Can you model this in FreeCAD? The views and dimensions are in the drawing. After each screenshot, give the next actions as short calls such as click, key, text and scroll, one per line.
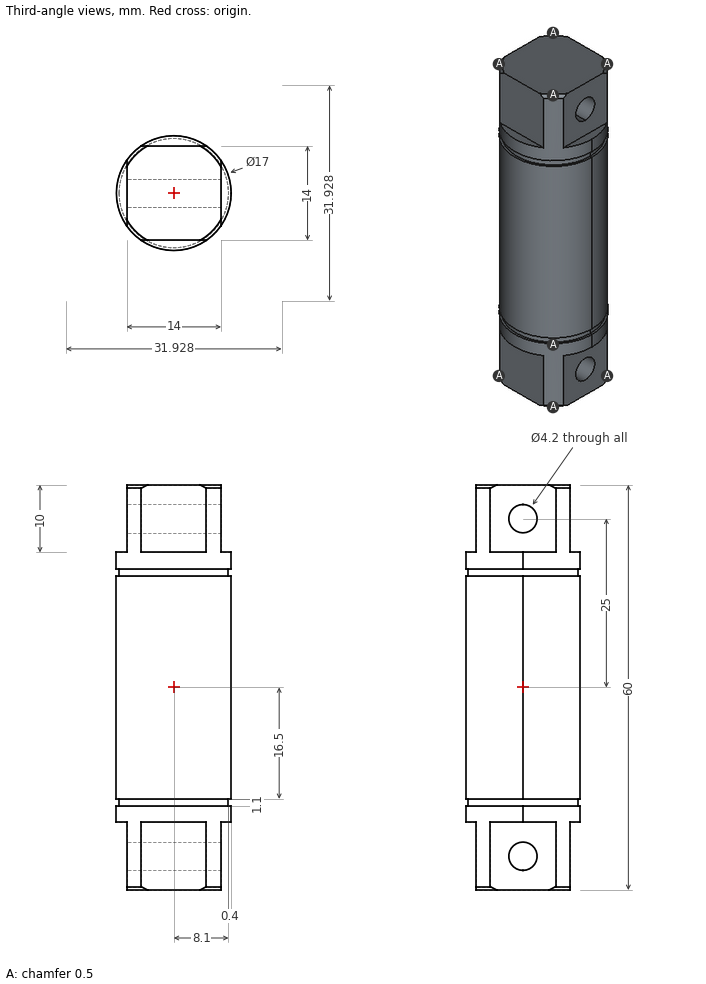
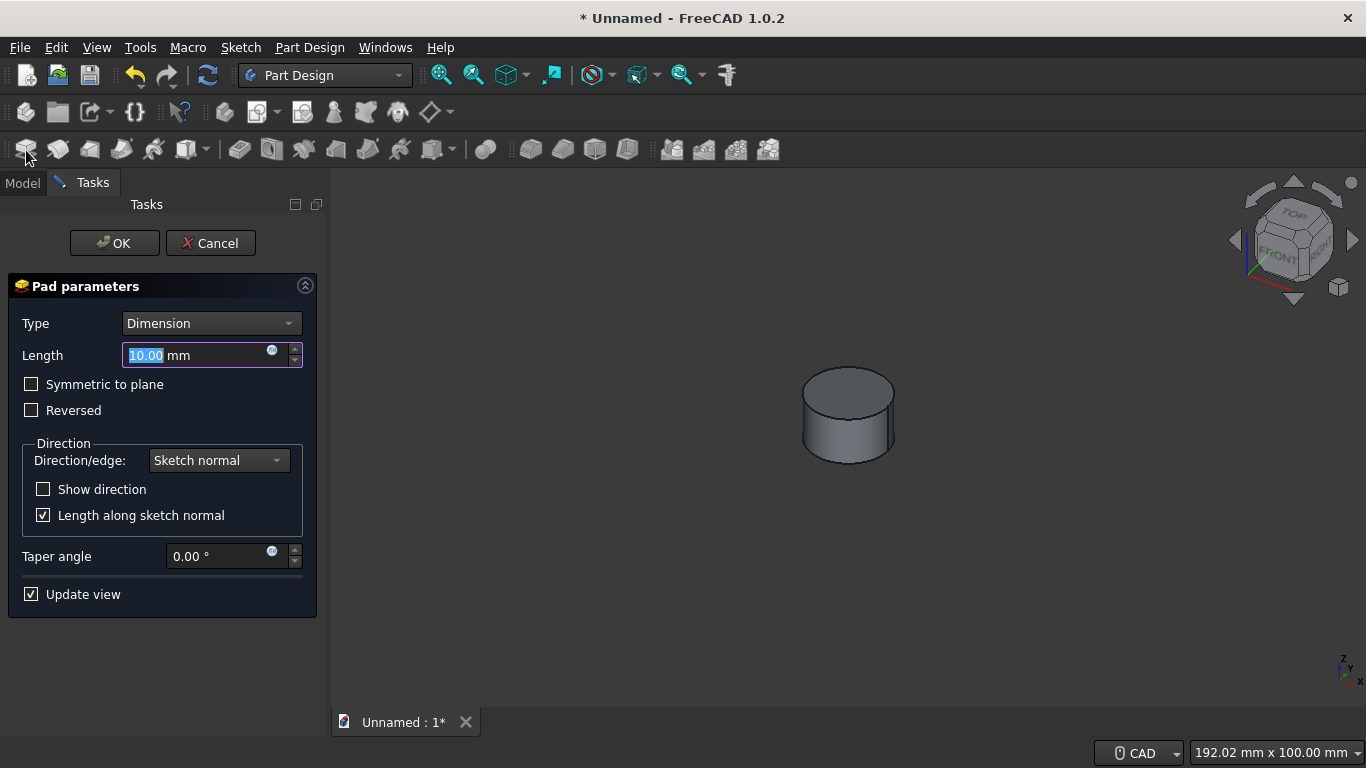
text(60)
key(Tab)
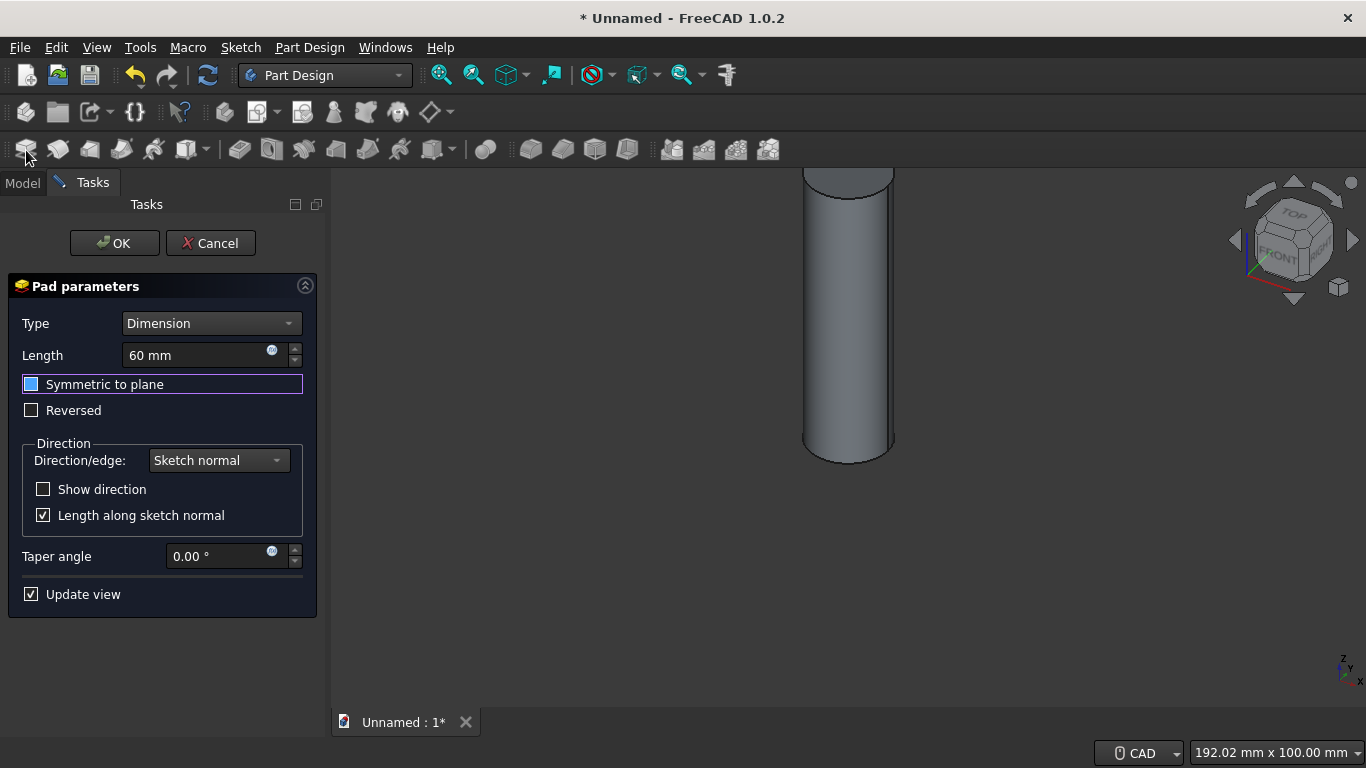
click(30, 384)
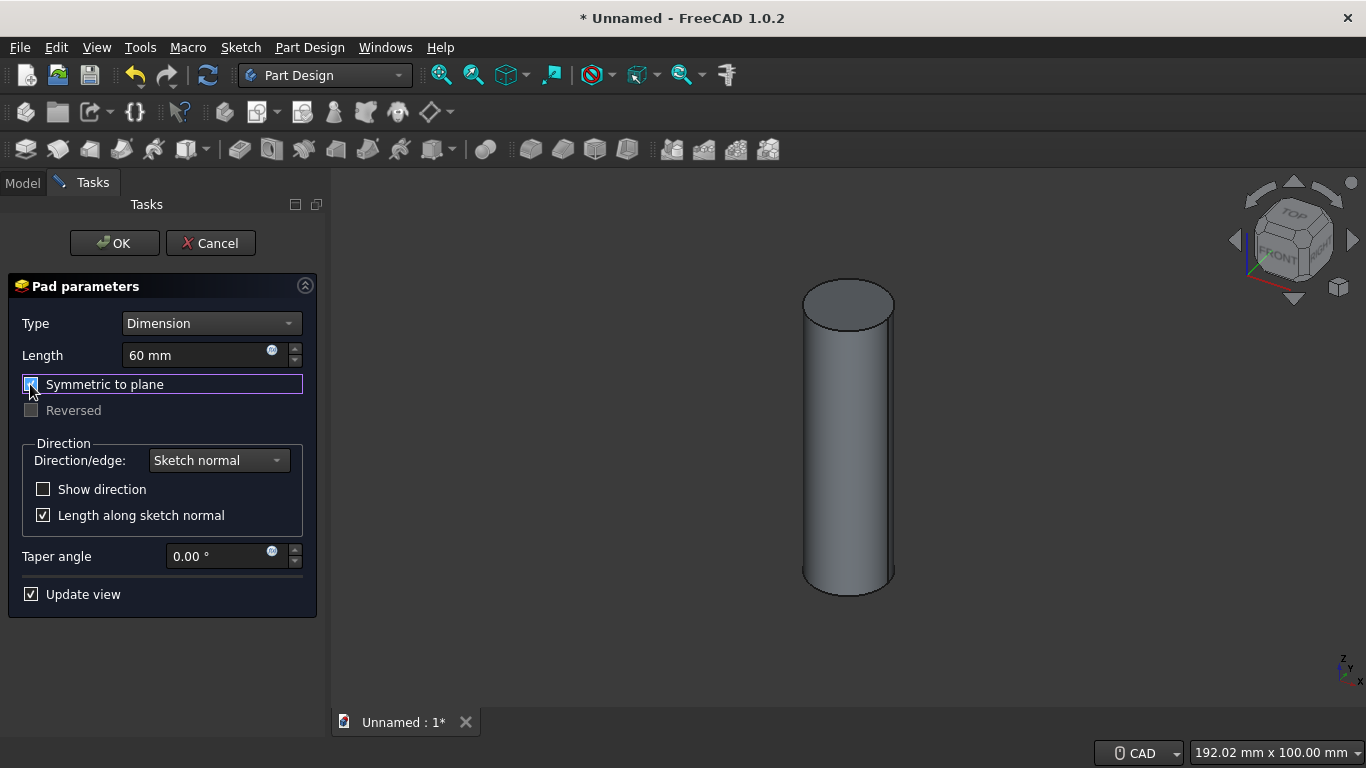
click(115, 243)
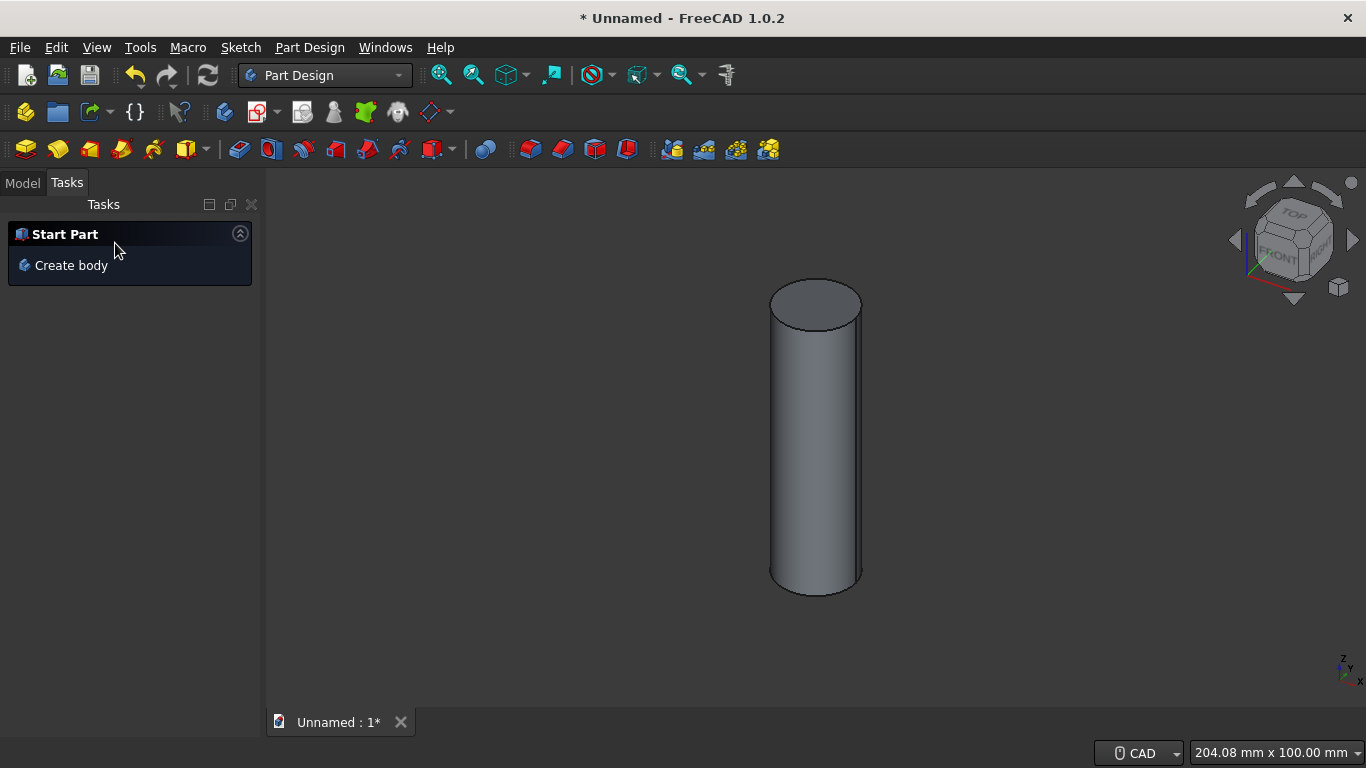
click(816, 304)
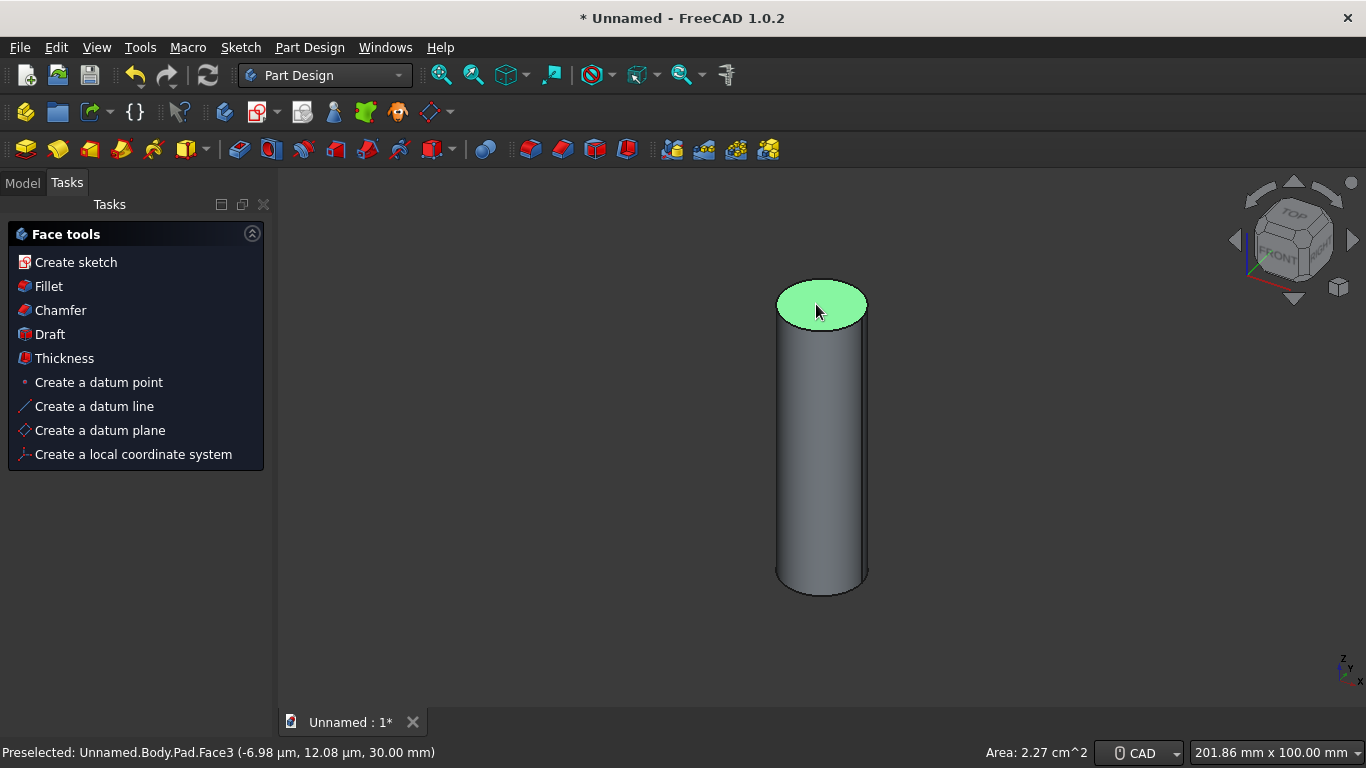
click(258, 112)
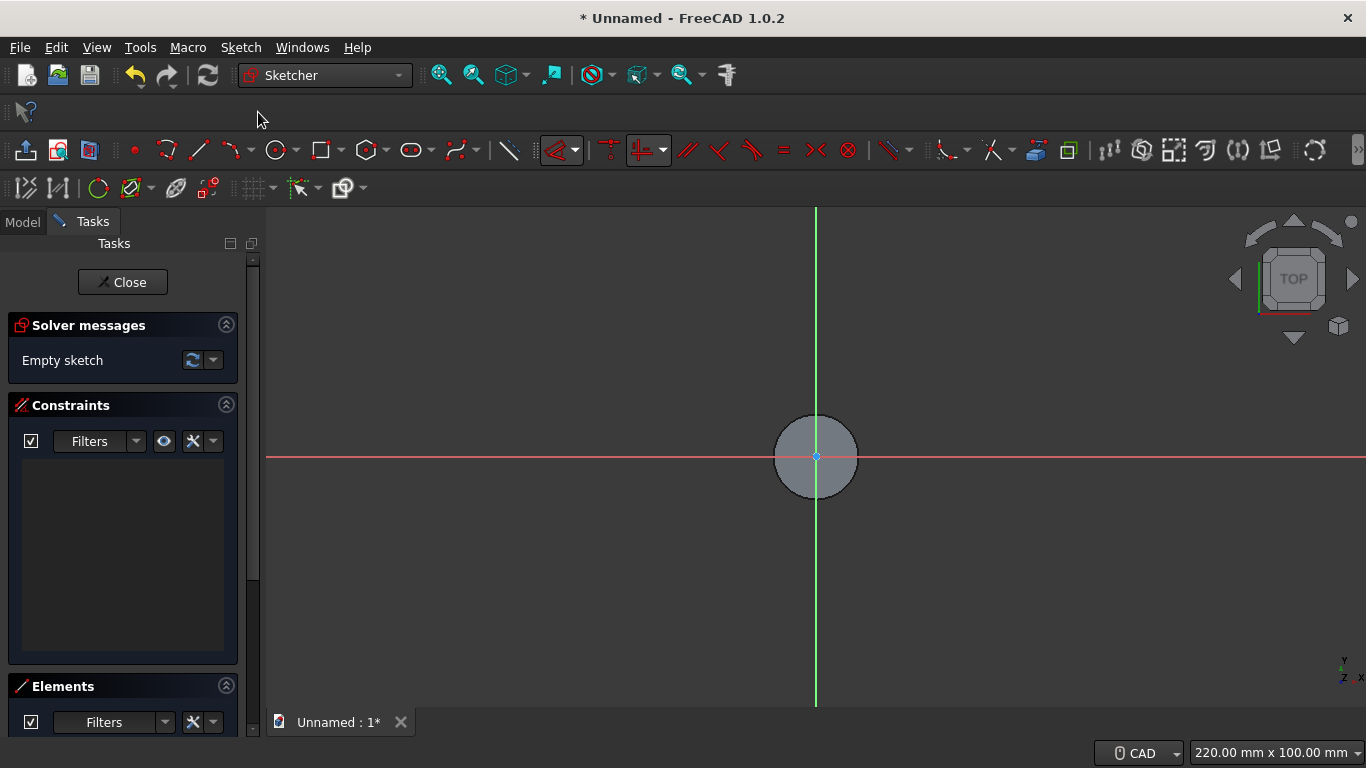
scroll(899, 457, up, 3)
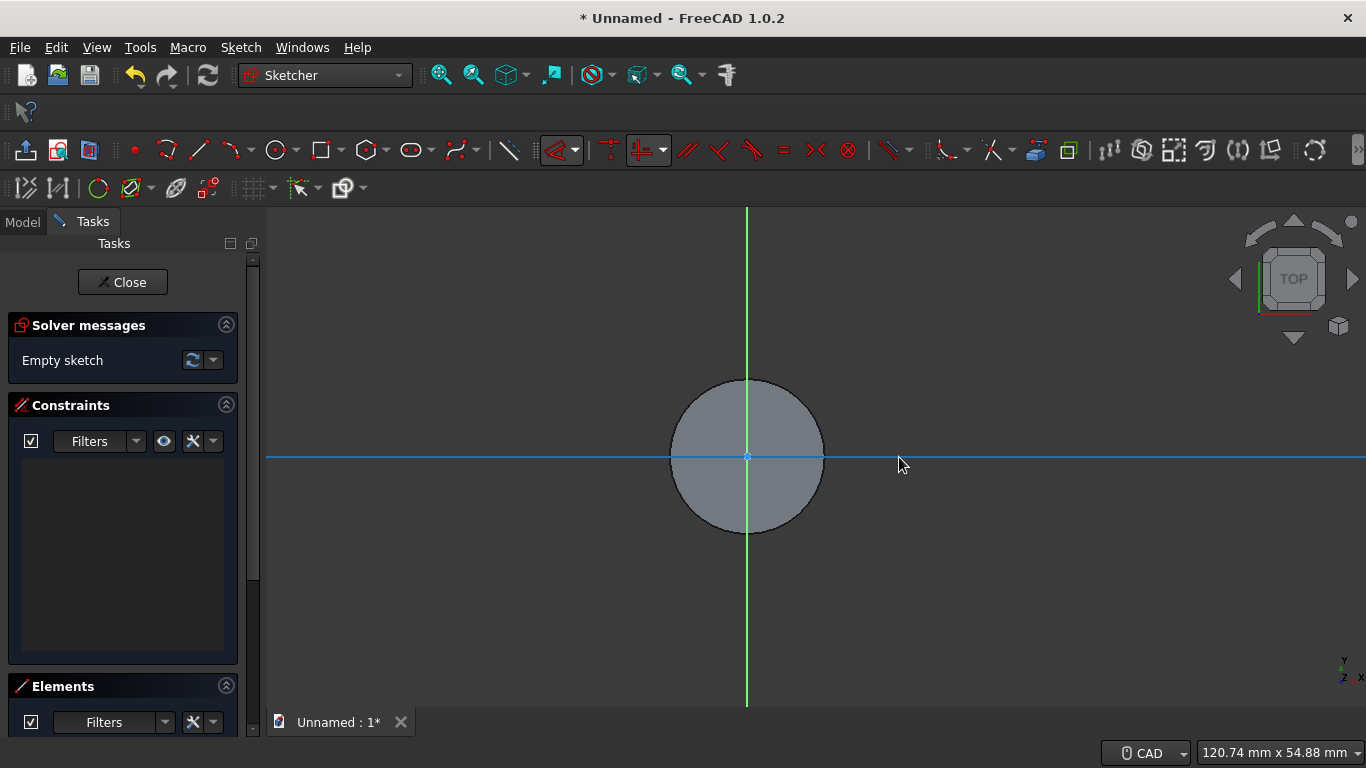
click(344, 150)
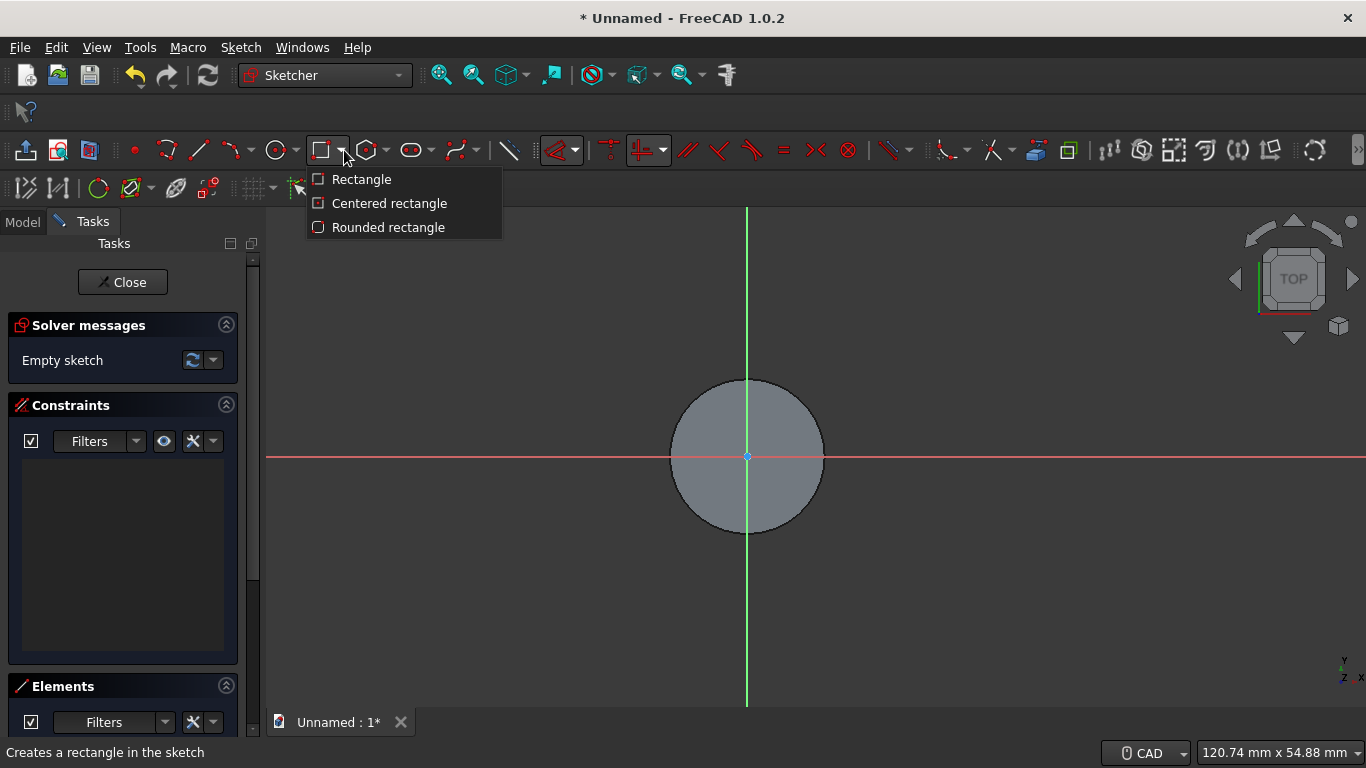
click(404, 203)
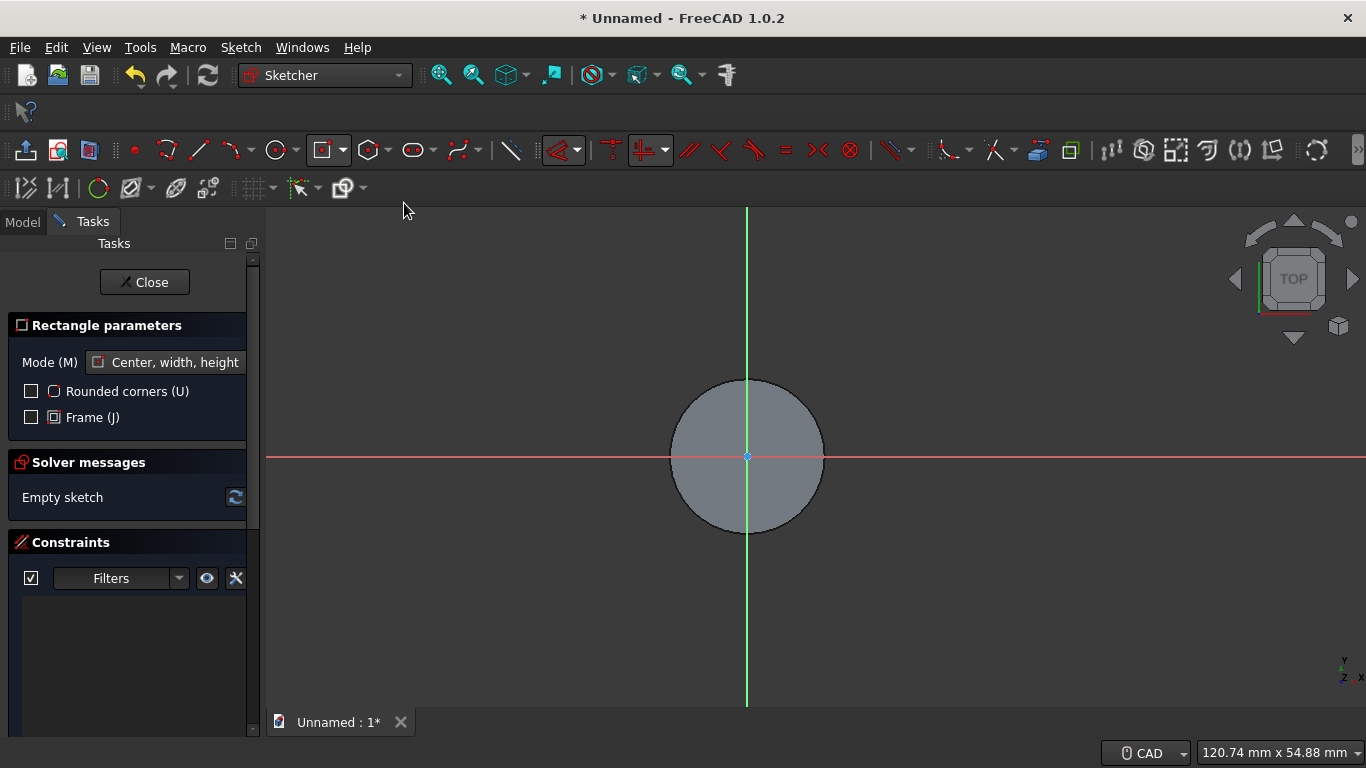
click(747, 457)
move(893, 311)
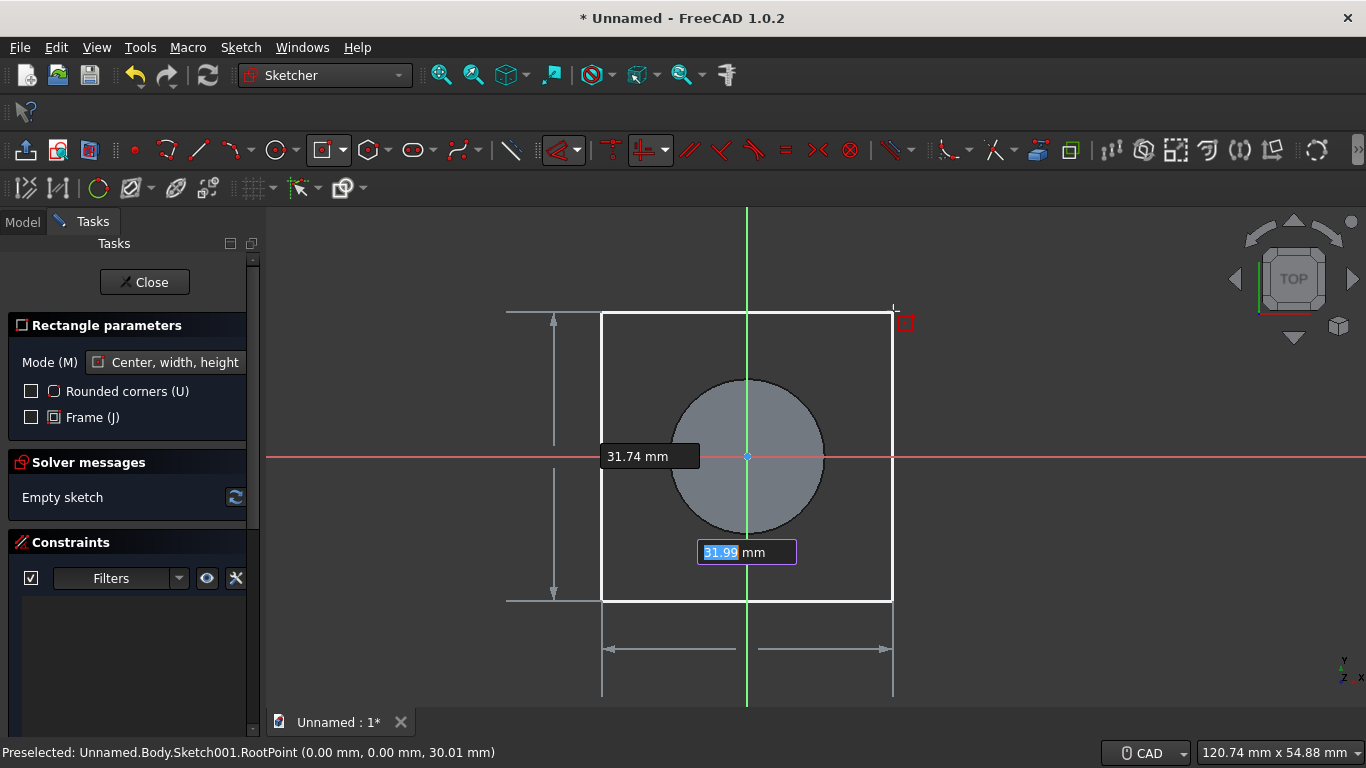
text(31.928)
key(Tab)
text(31.928)
key(Return)